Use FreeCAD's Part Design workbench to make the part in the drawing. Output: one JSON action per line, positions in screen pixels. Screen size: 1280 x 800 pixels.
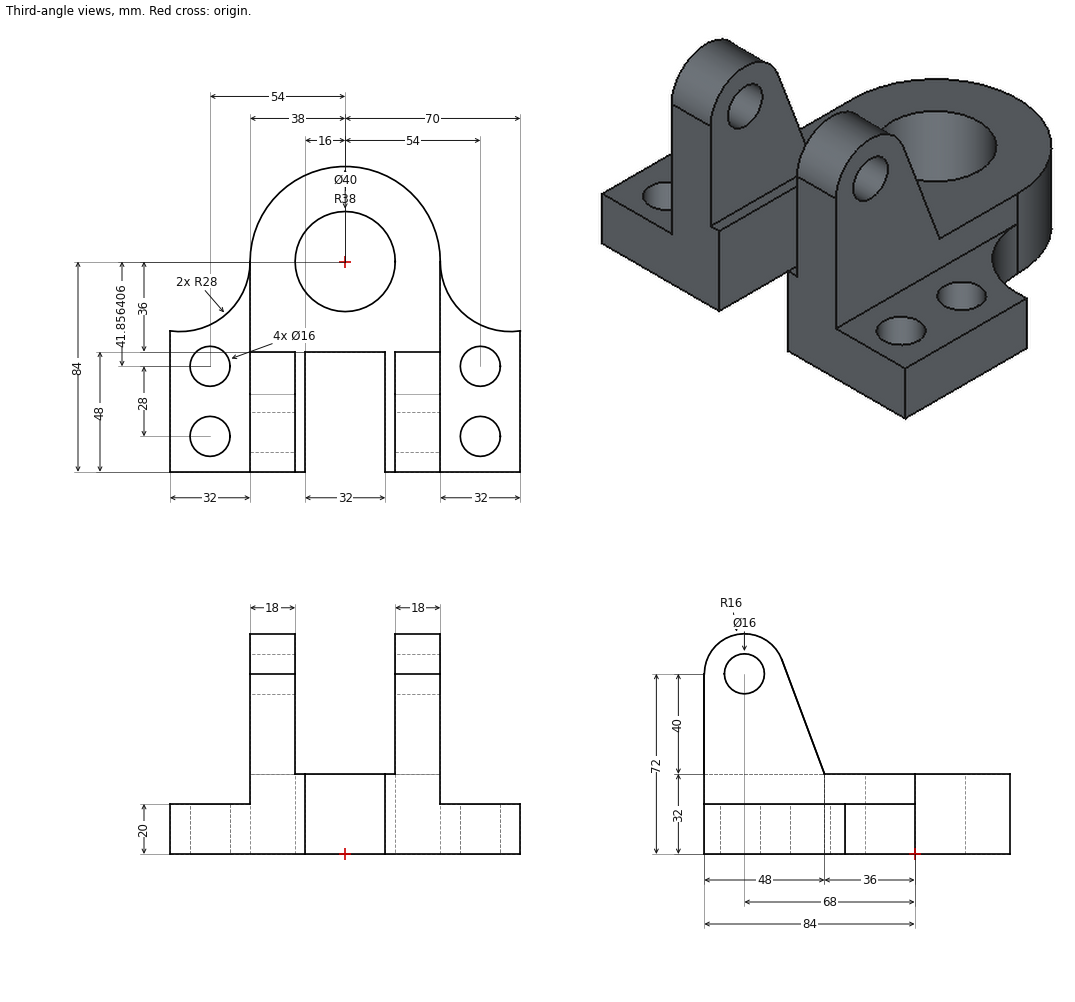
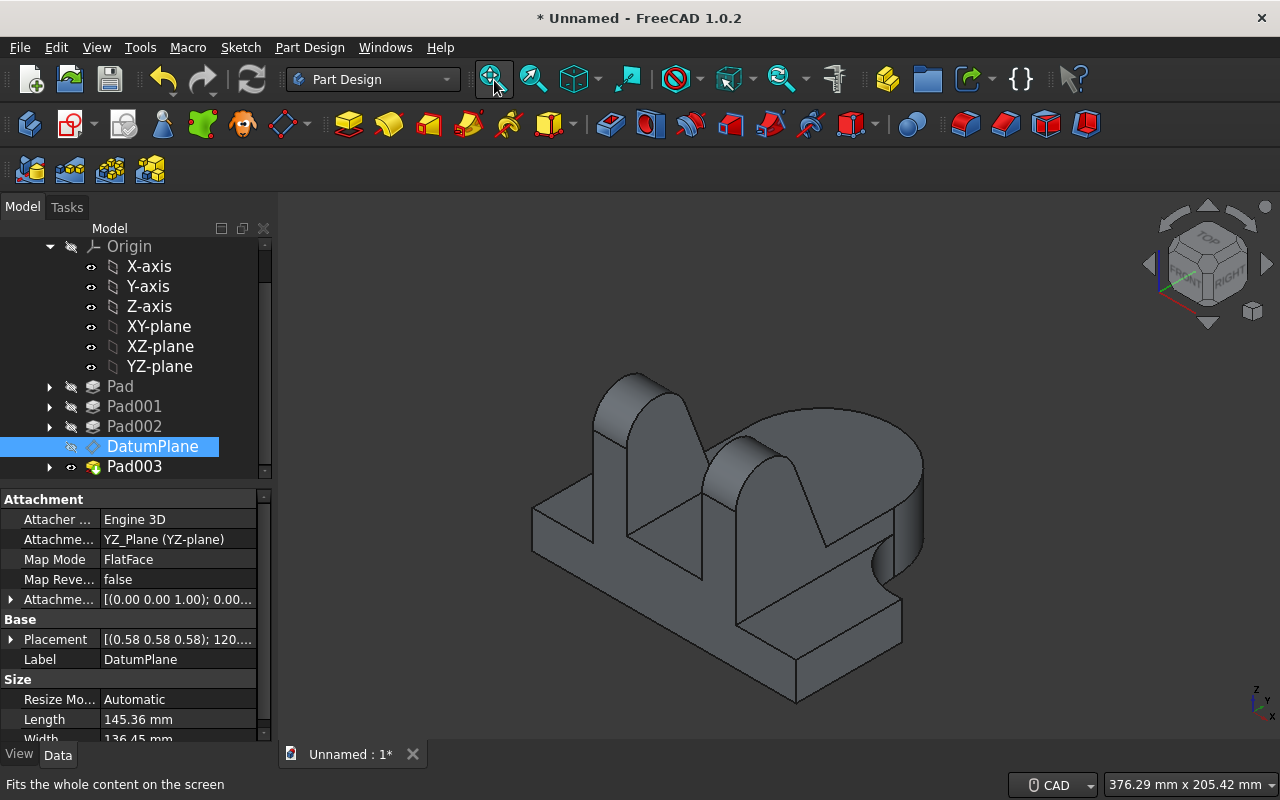
{"action": "left_click", "coordinate": [812, 472]}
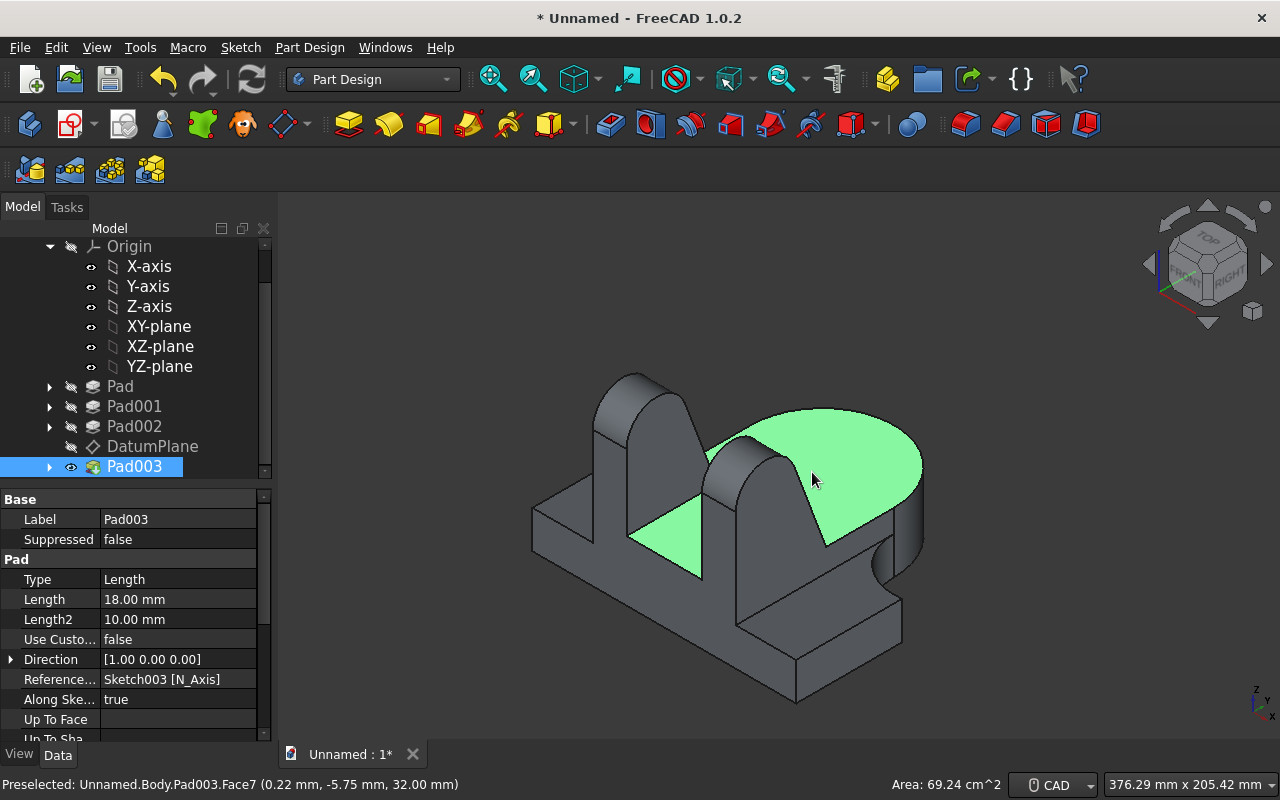
{"action": "left_click", "coordinate": [70, 124]}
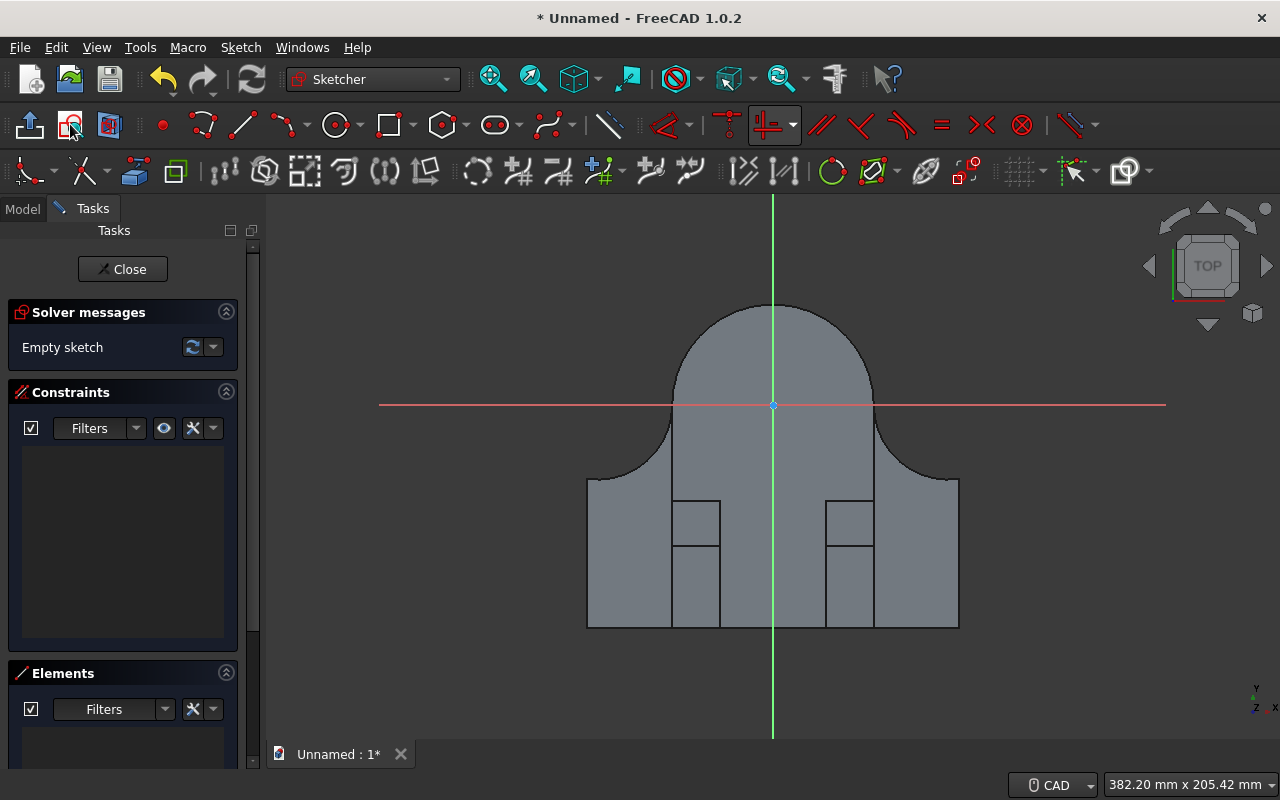
{"action": "left_click", "coordinate": [110, 126]}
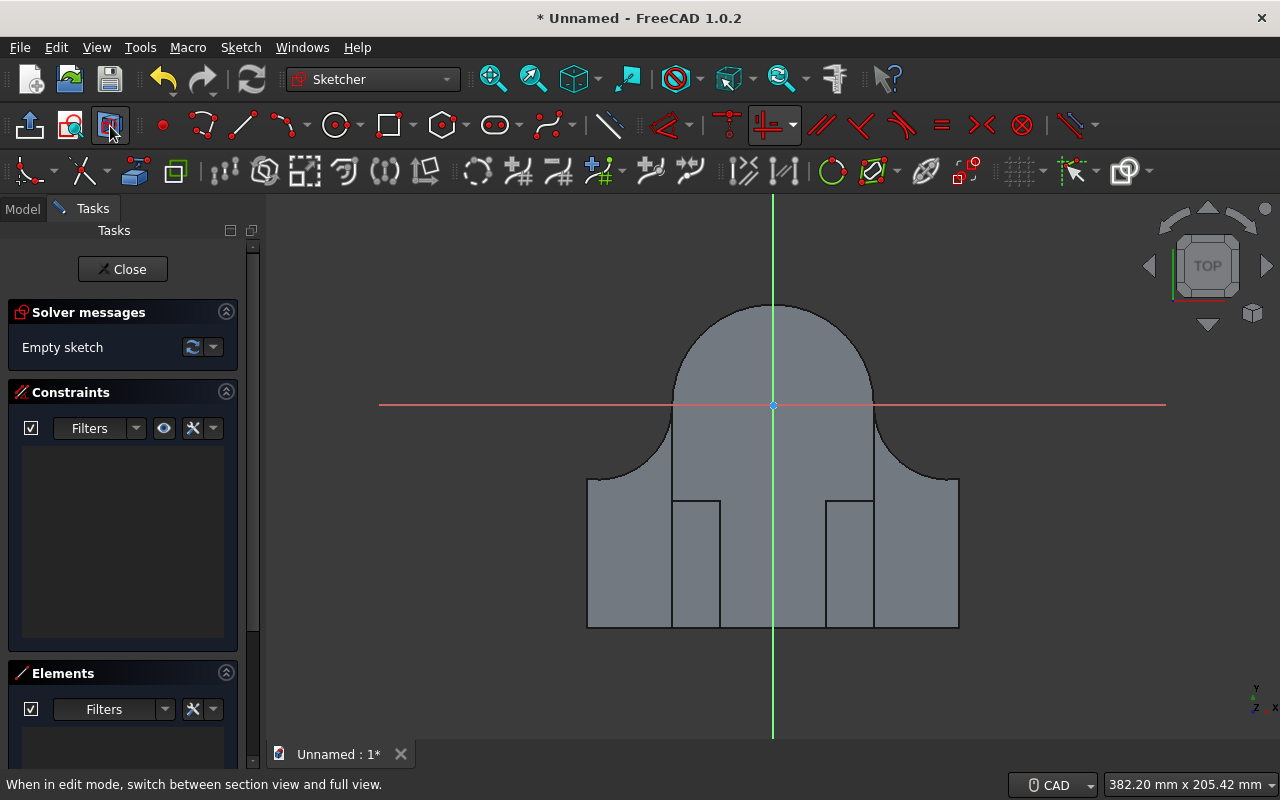
{"action": "scroll", "coordinate": [912, 619], "scroll_direction": "up", "scroll_amount": 2}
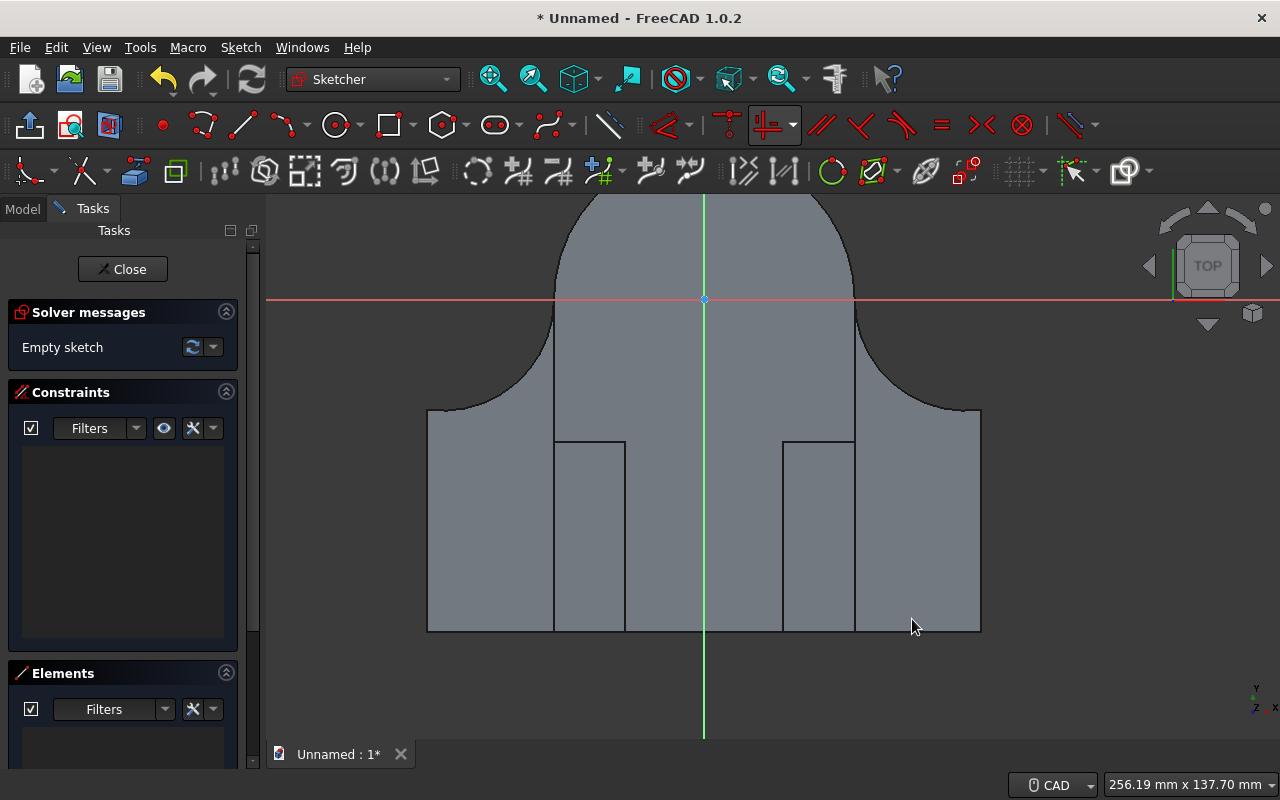
{"action": "left_click", "coordinate": [390, 126]}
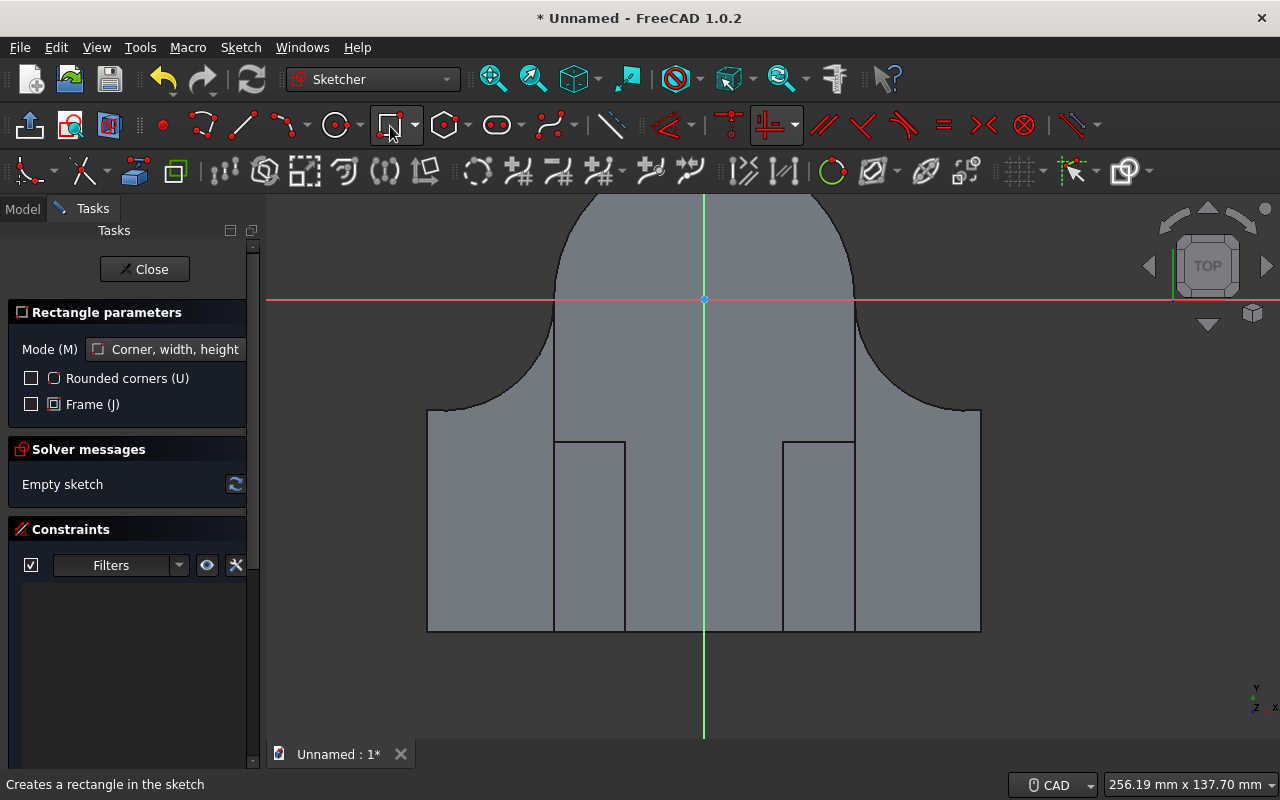
{"action": "left_click", "coordinate": [641, 442]}
{"action": "left_click", "coordinate": [768, 632]}
{"action": "key", "text": "Escape"}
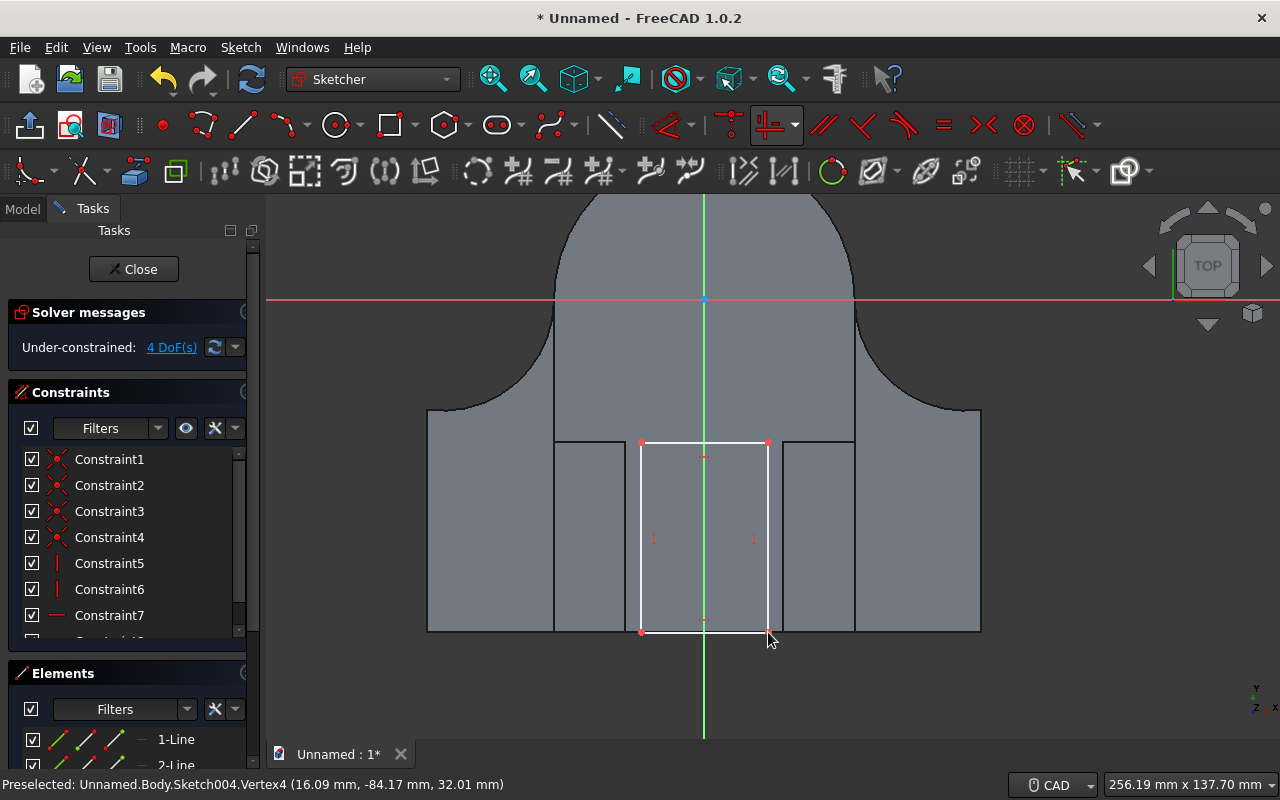
{"action": "left_click", "coordinate": [666, 126]}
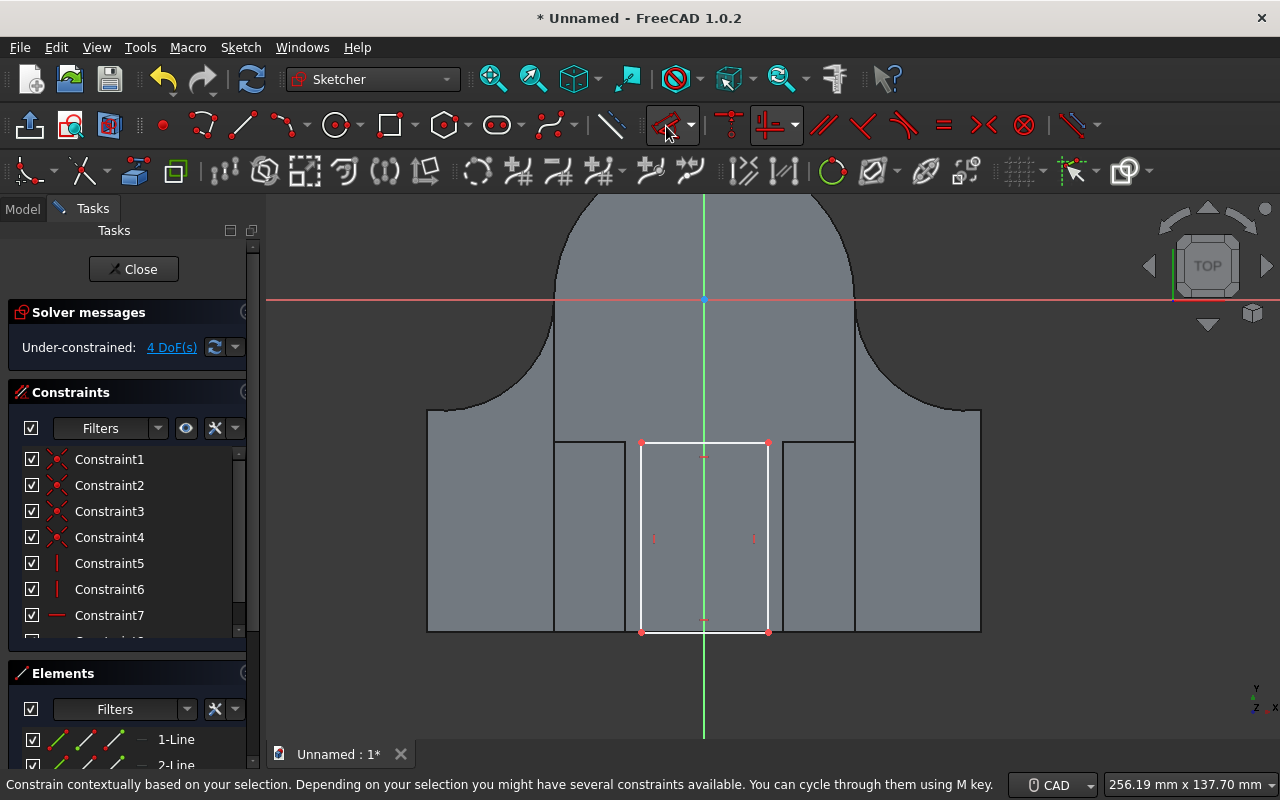
{"action": "left_click", "coordinate": [641, 500]}
{"action": "left_click", "coordinate": [607, 538]}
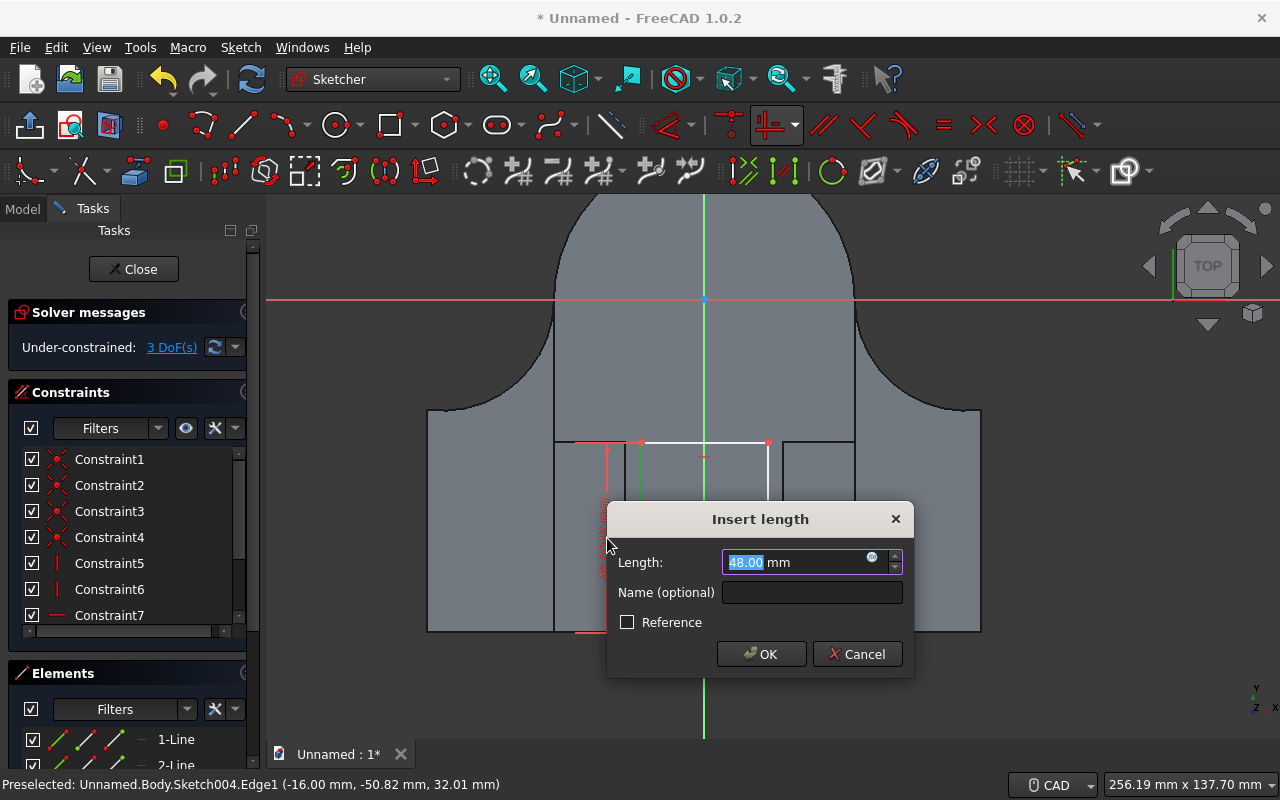
{"action": "type", "text": "48"}
{"action": "key", "text": "Return"}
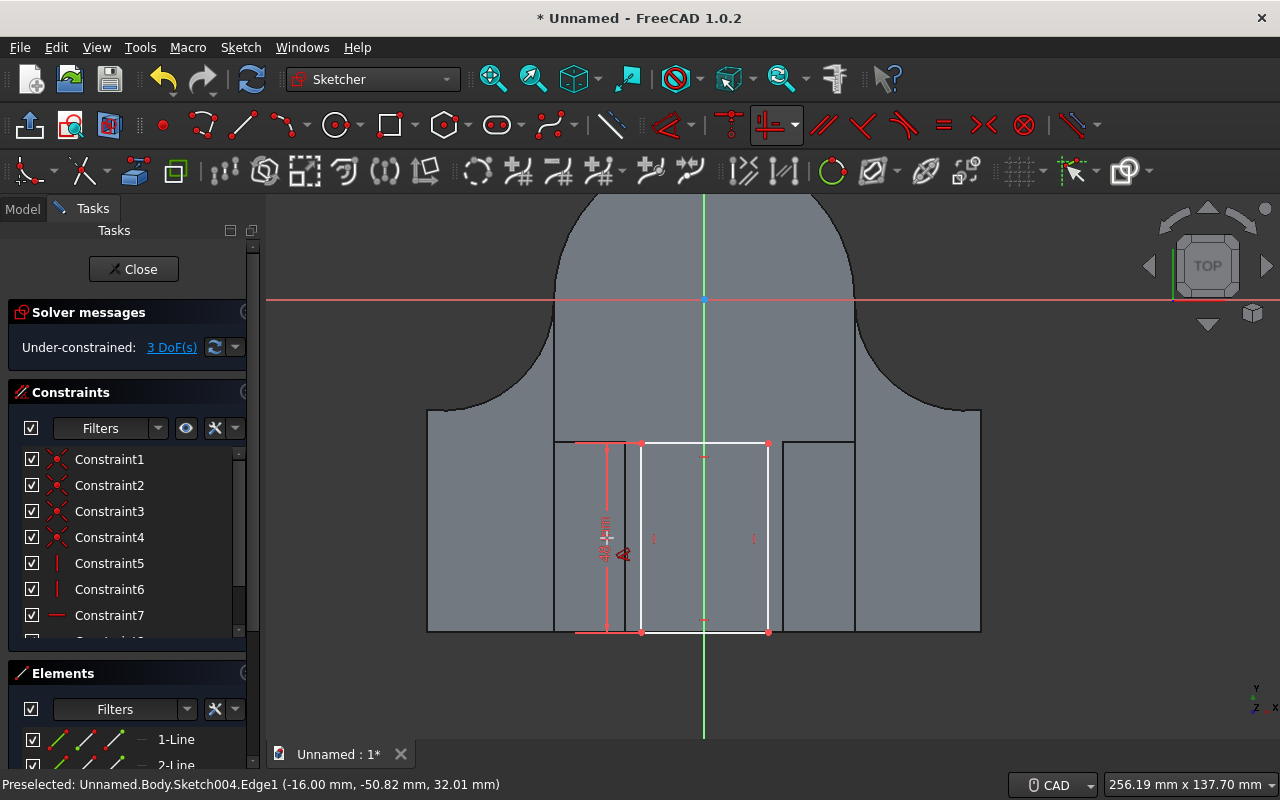
{"action": "left_click", "coordinate": [679, 633]}
{"action": "left_click", "coordinate": [675, 667]}